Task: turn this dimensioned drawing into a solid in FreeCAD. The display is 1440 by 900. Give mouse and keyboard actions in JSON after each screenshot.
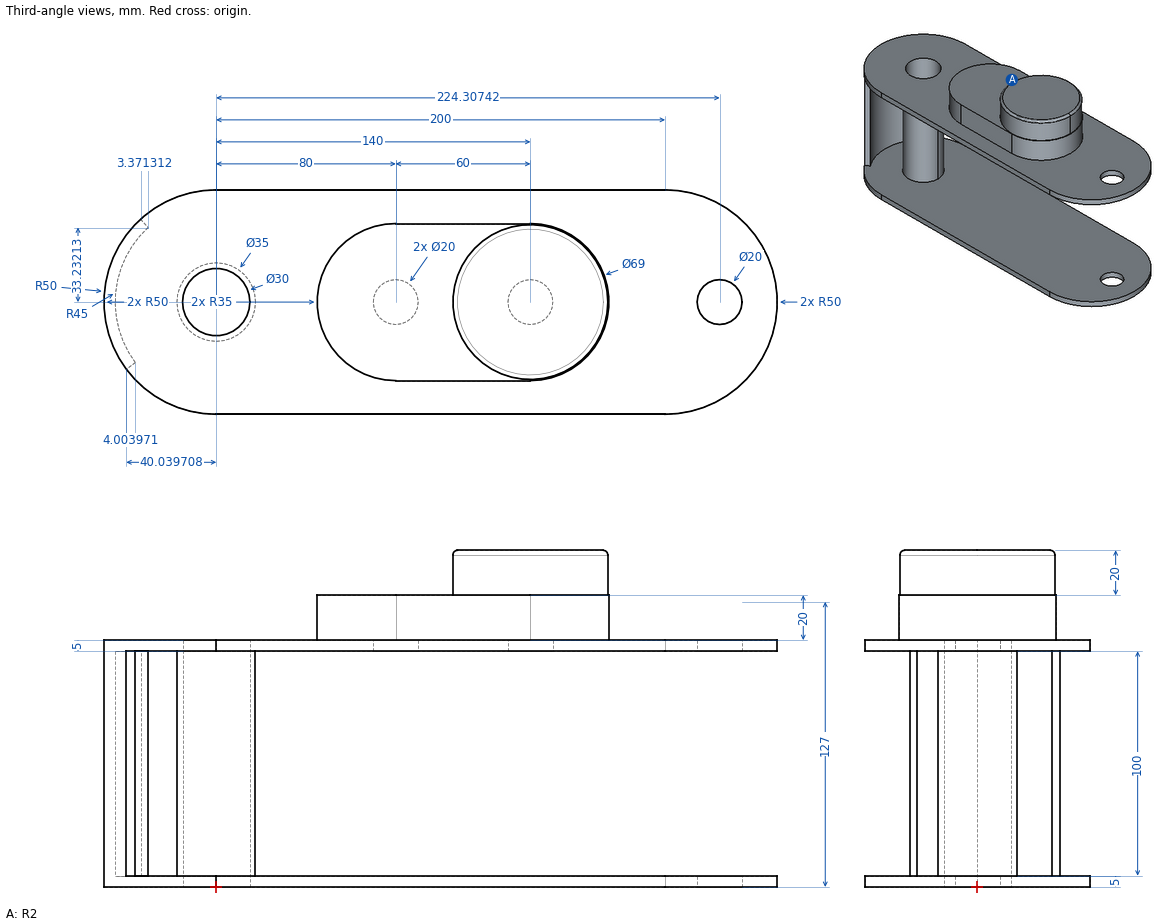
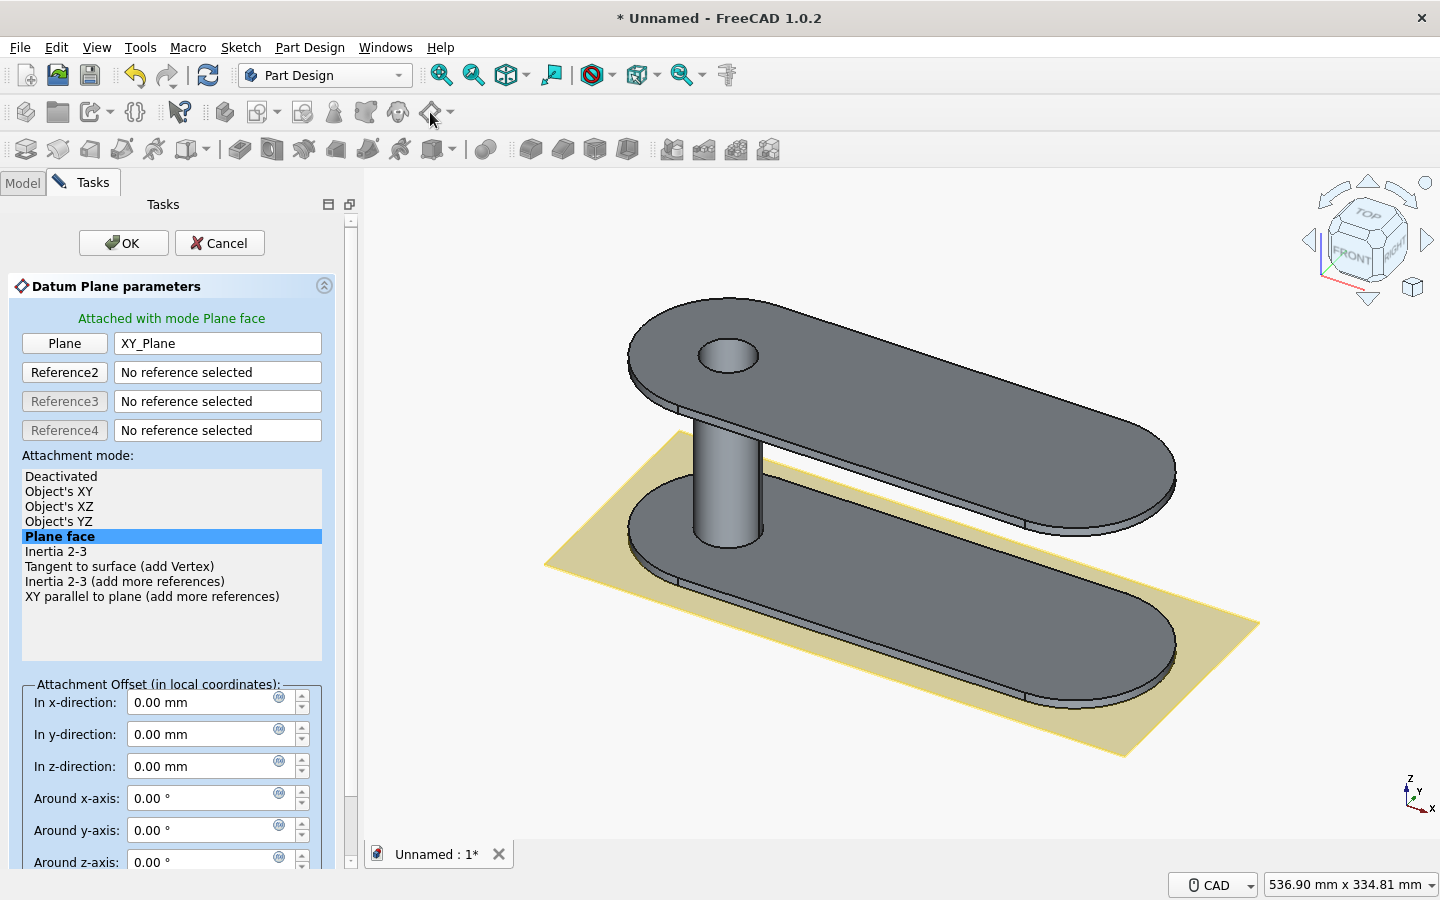
{"action": "triple_click", "coordinate": [210, 766]}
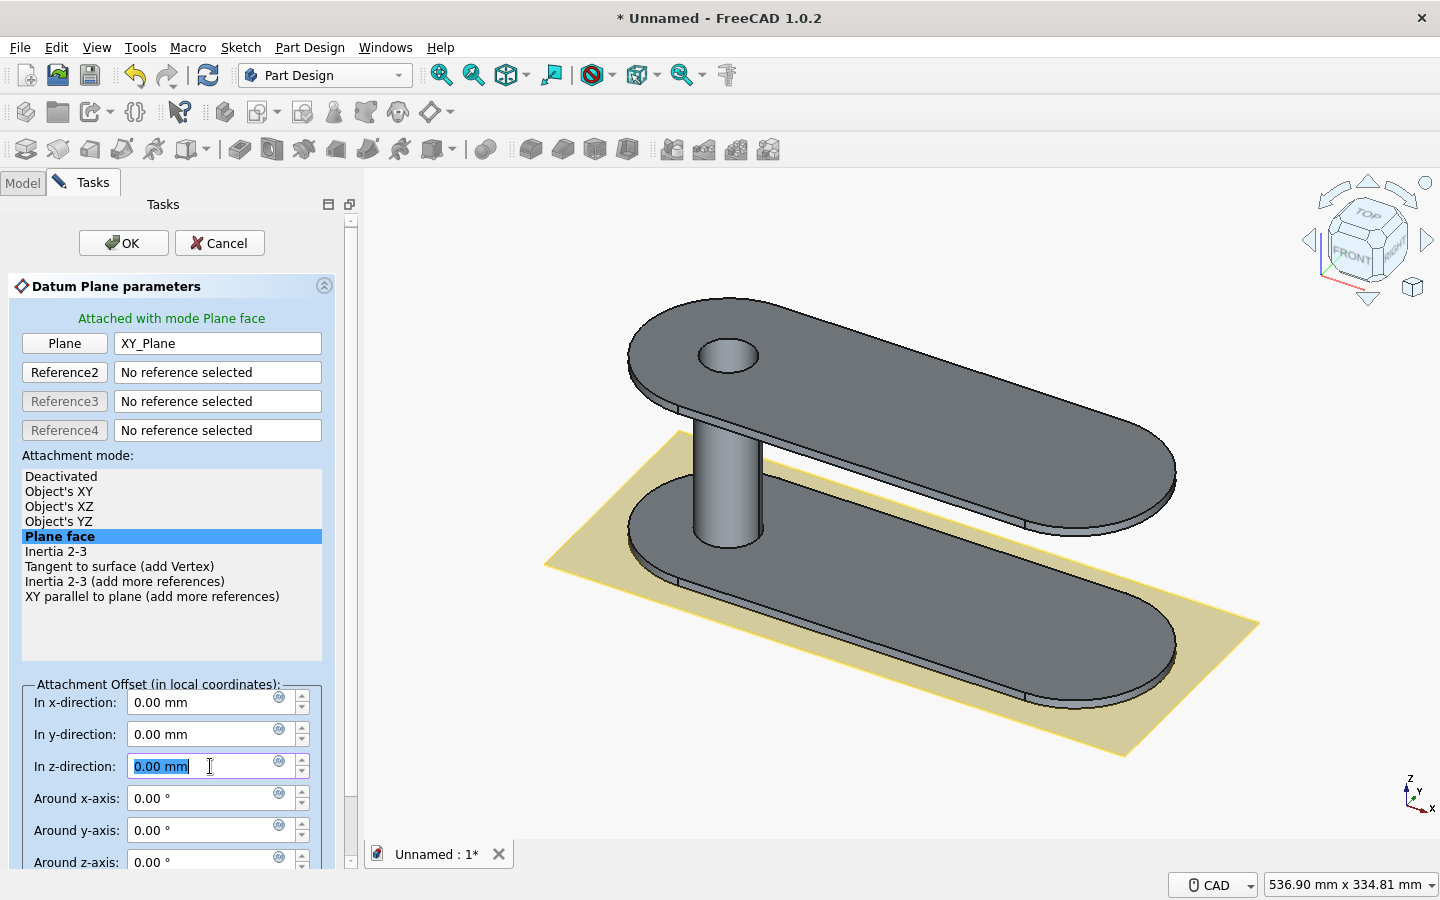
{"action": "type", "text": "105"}
{"action": "key", "text": "Tab"}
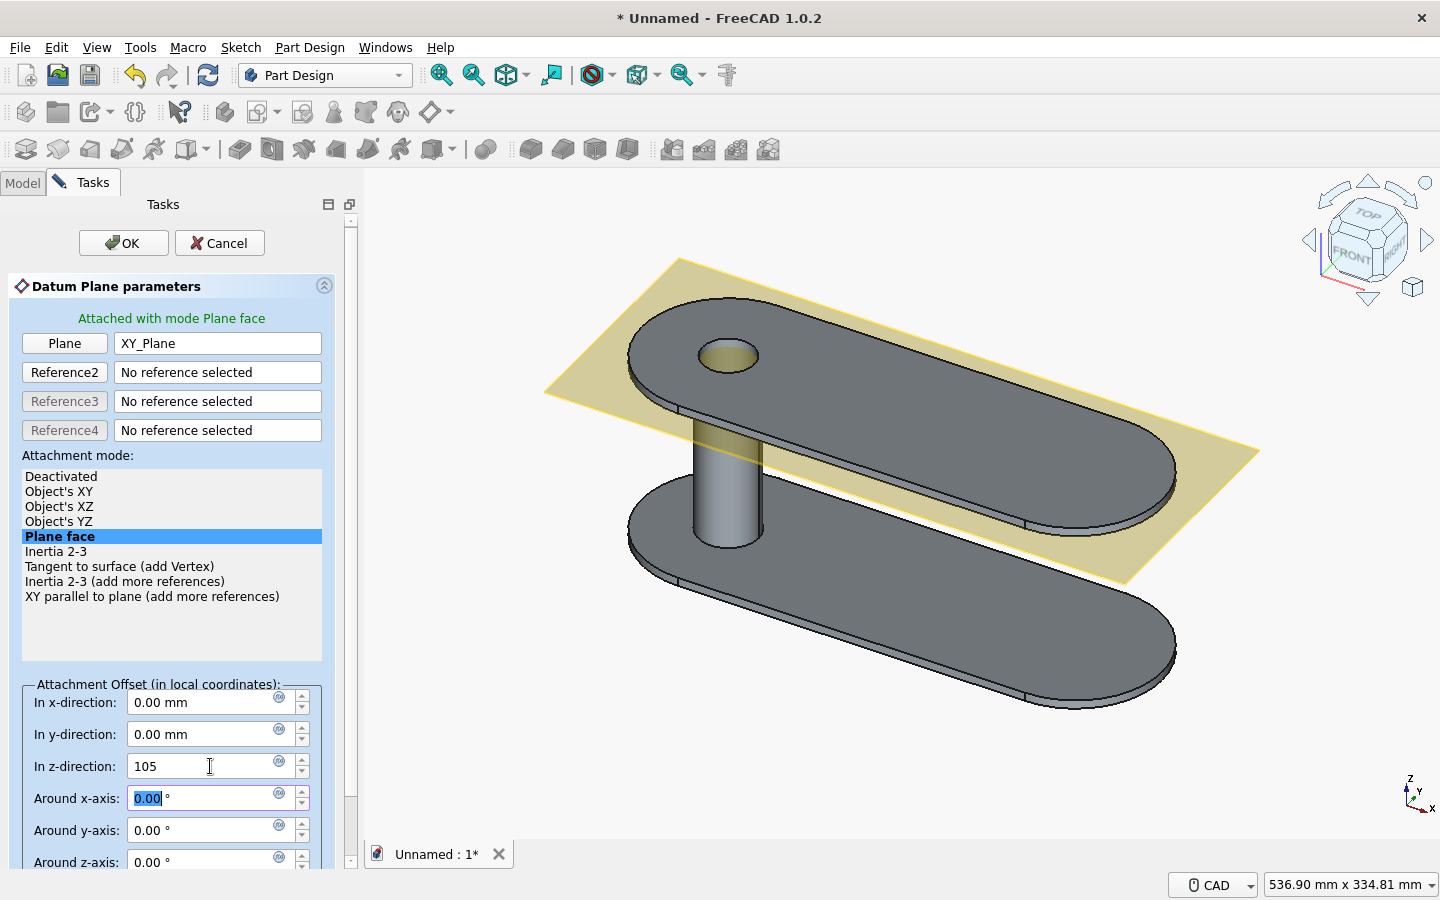
{"action": "left_click", "coordinate": [124, 243]}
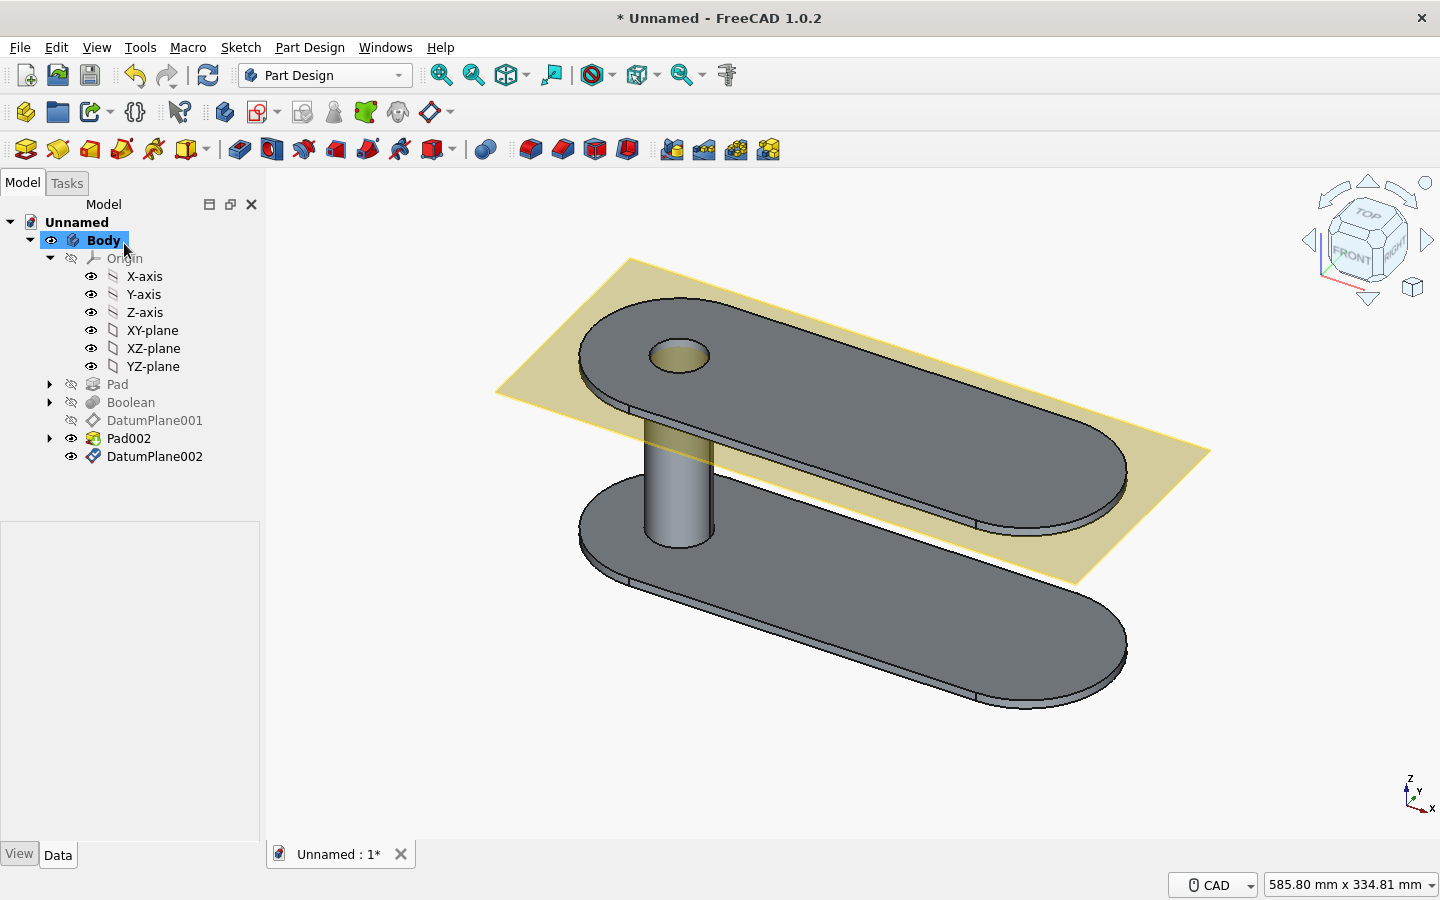
{"action": "left_click", "coordinate": [116, 456]}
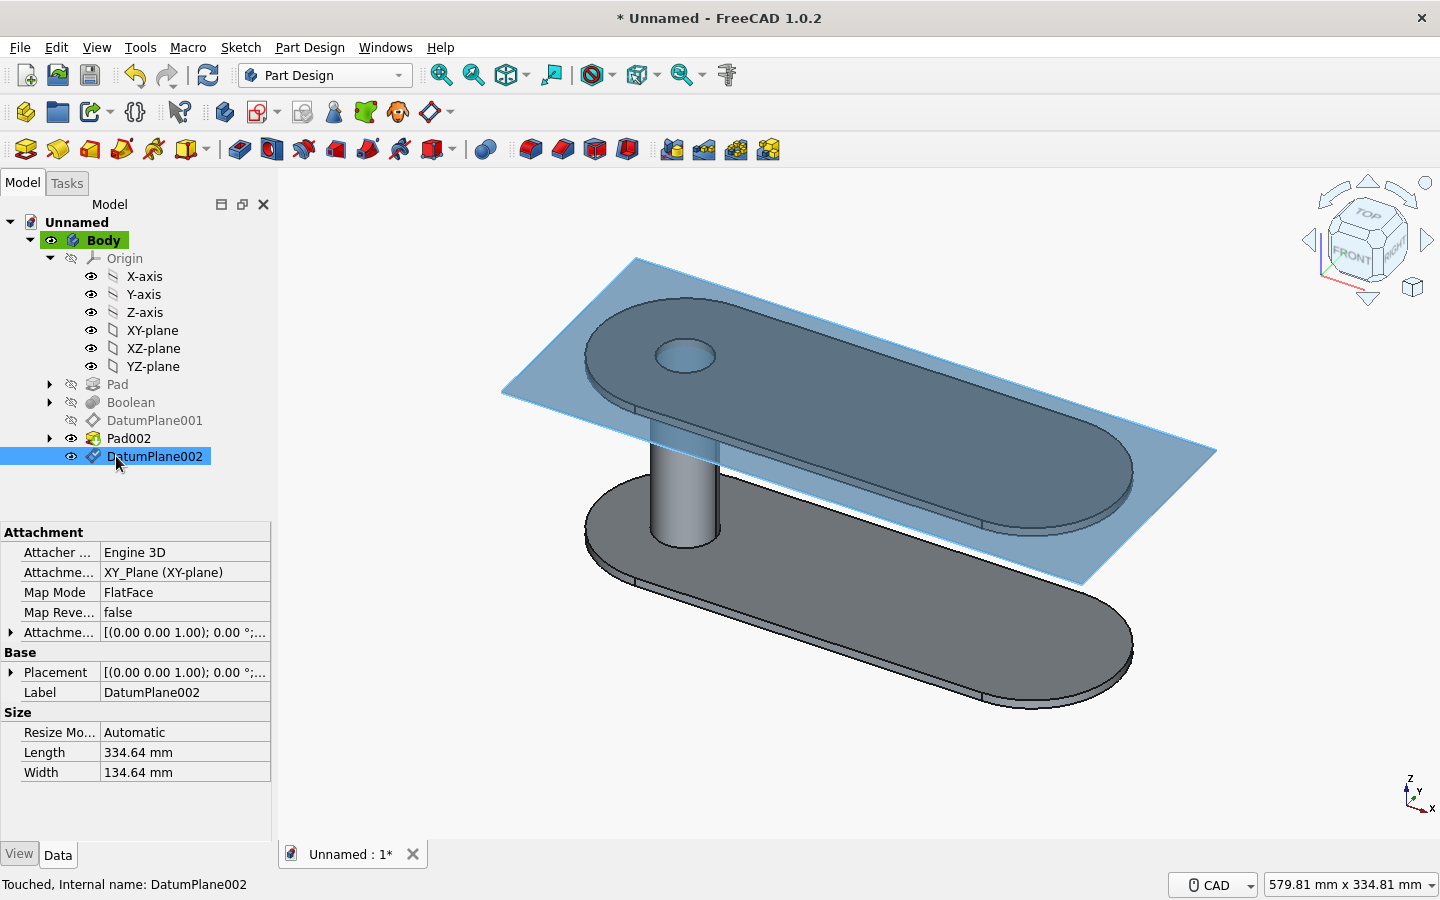
{"action": "left_click", "coordinate": [258, 112]}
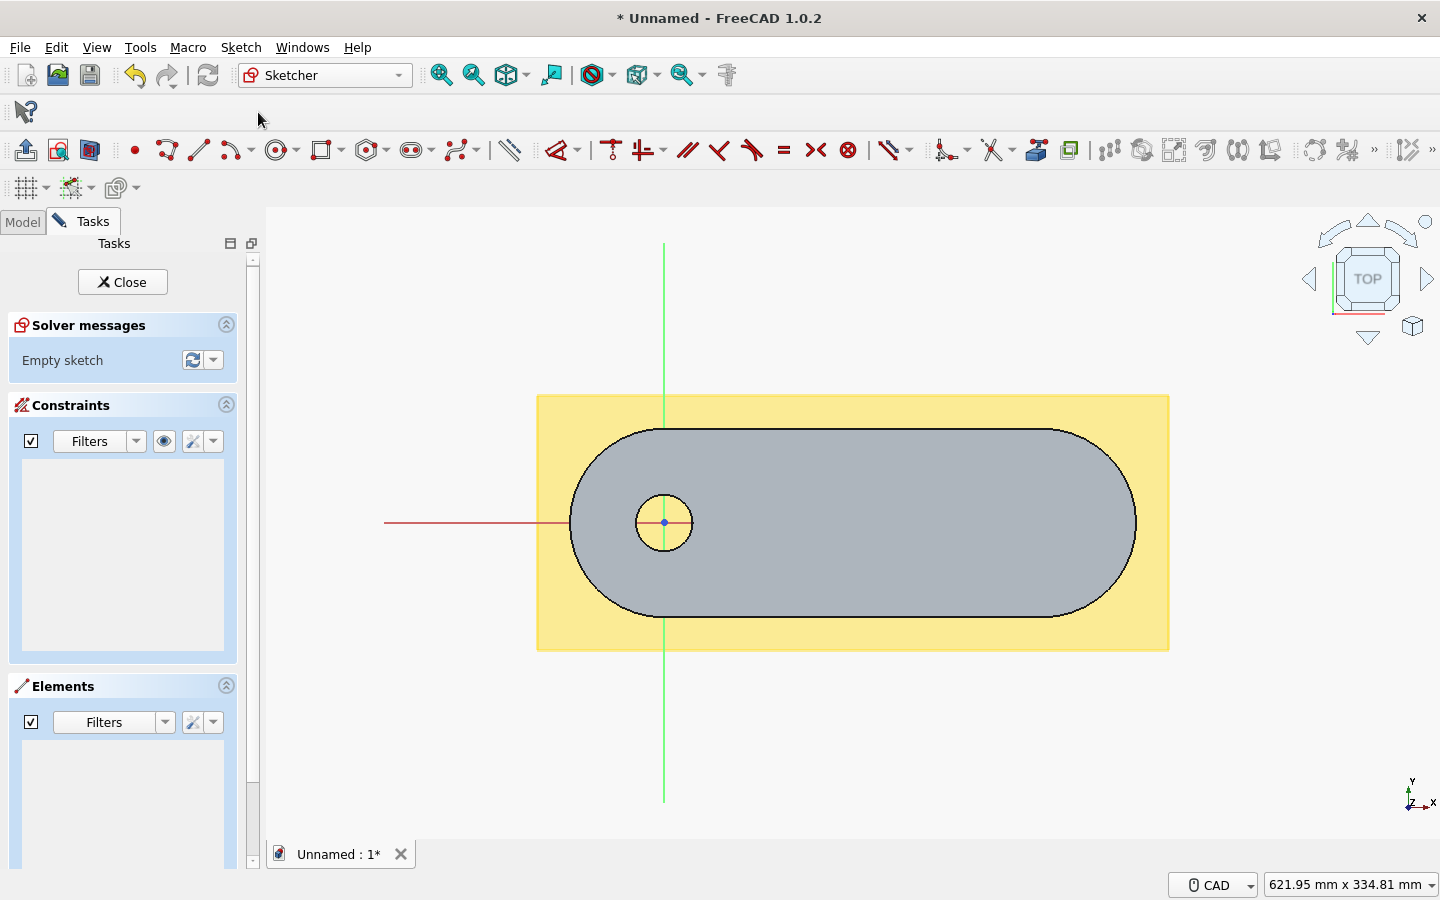
{"action": "left_click", "coordinate": [90, 150]}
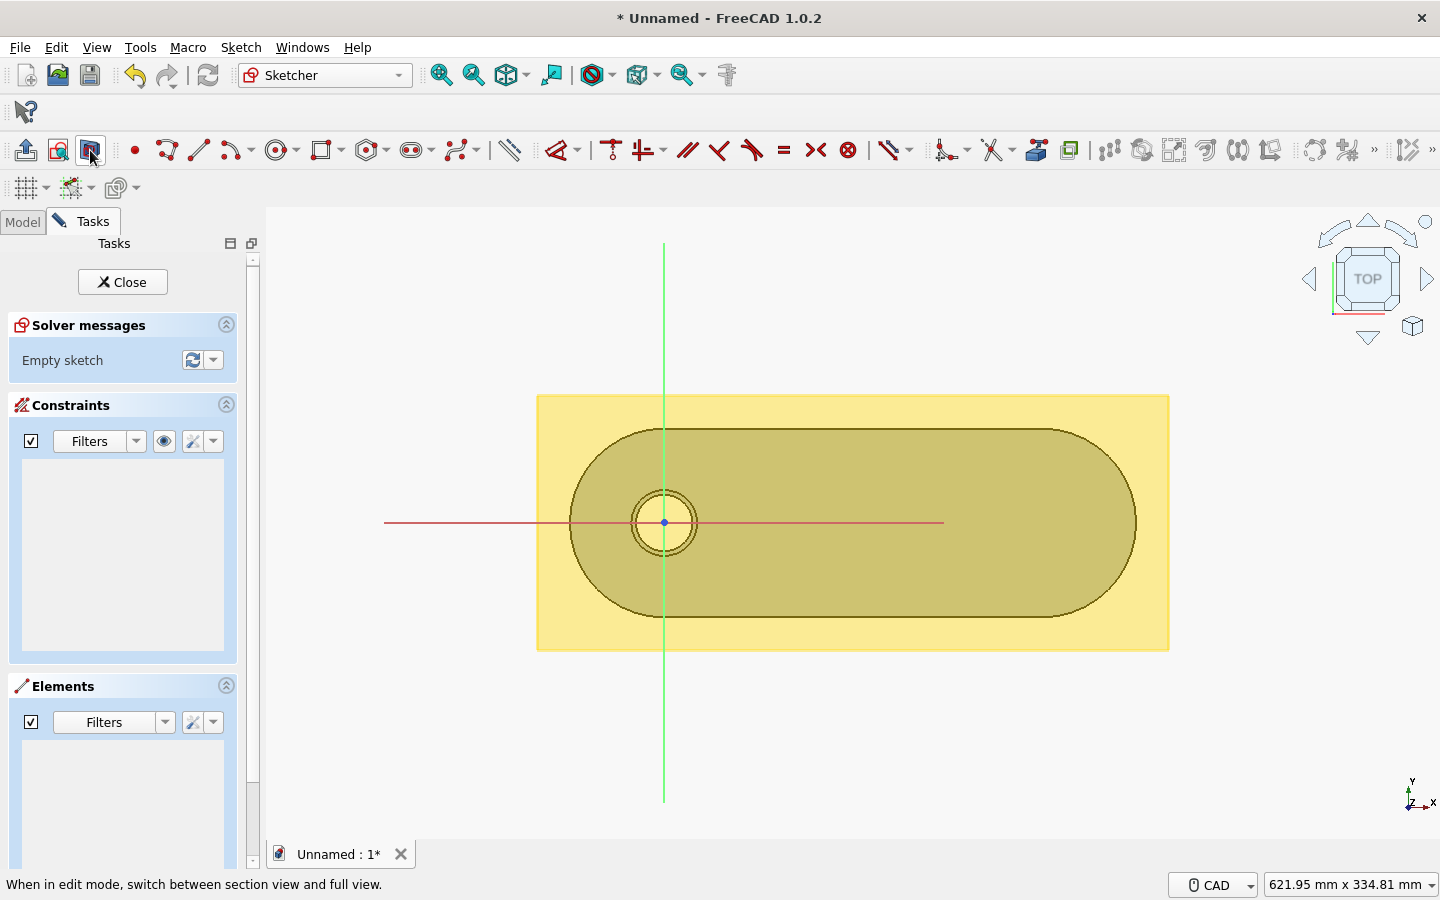
{"action": "scroll", "coordinate": [823, 523], "scroll_direction": "up", "scroll_amount": 4}